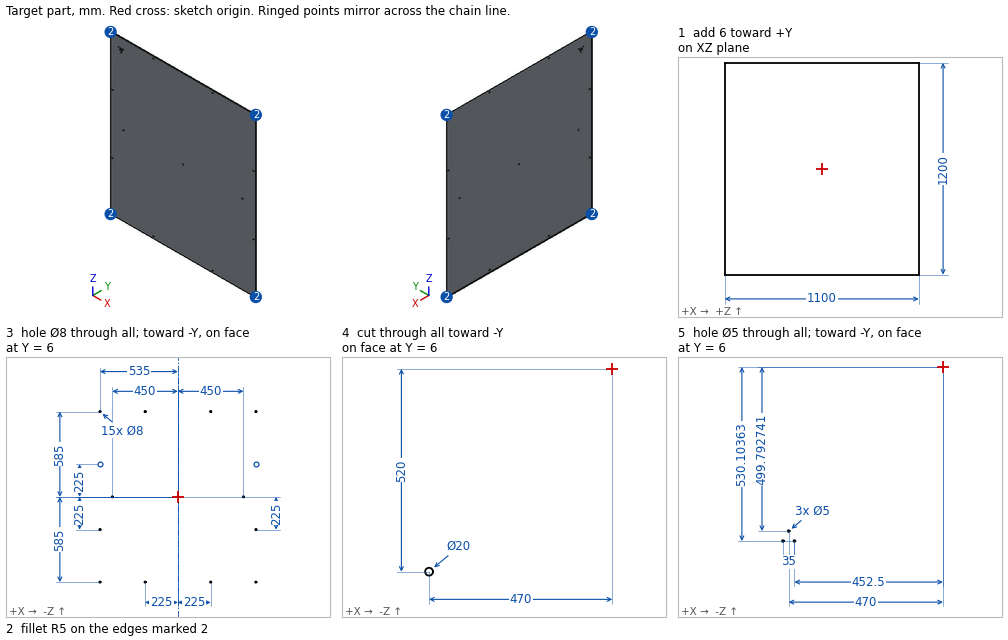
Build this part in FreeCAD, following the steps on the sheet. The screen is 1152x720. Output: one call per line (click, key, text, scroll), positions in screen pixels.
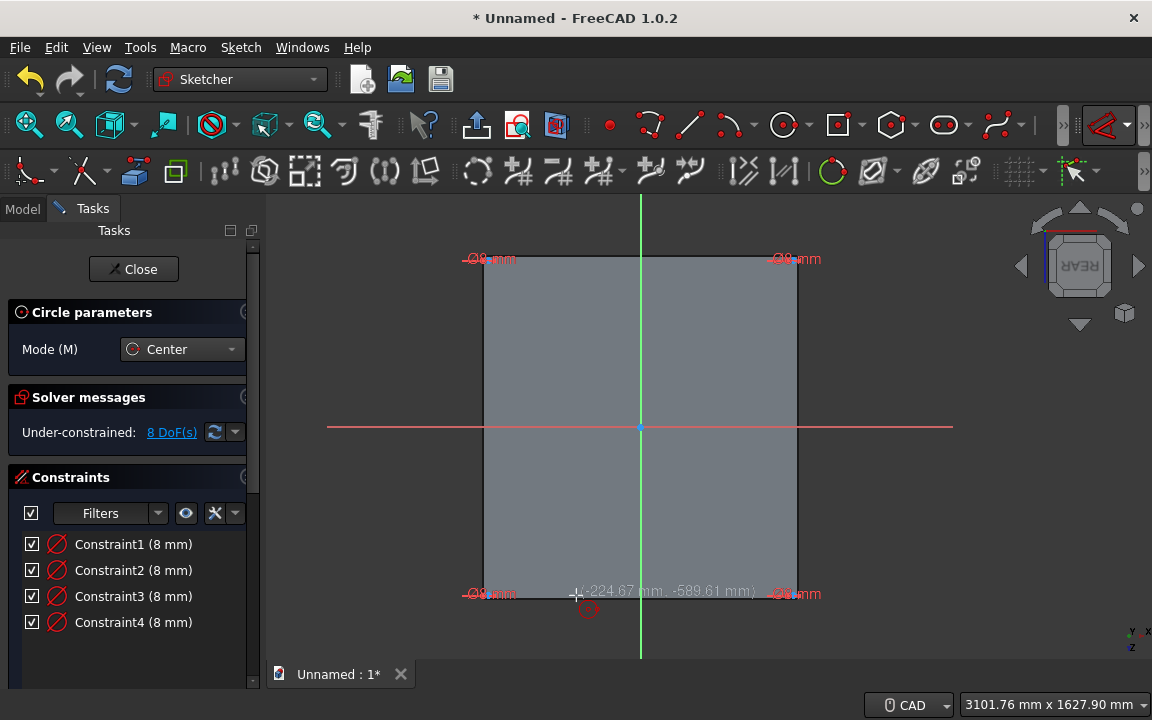
click(576, 595)
move(577, 594)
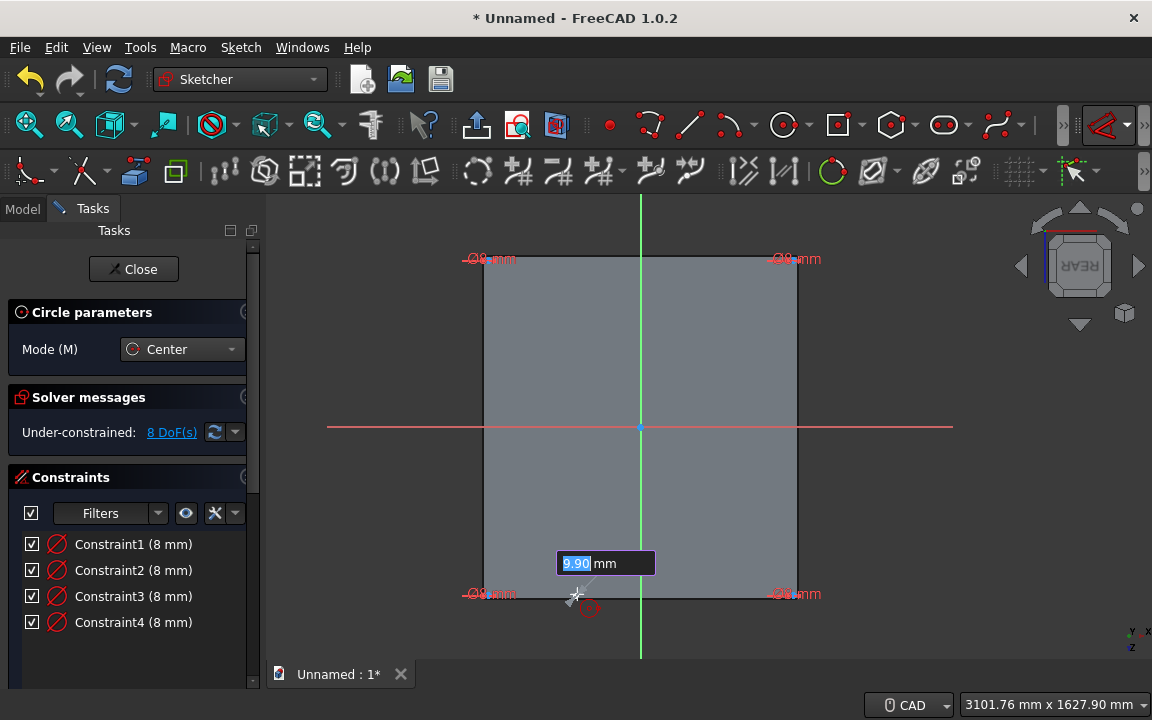
text(8)
key(Return)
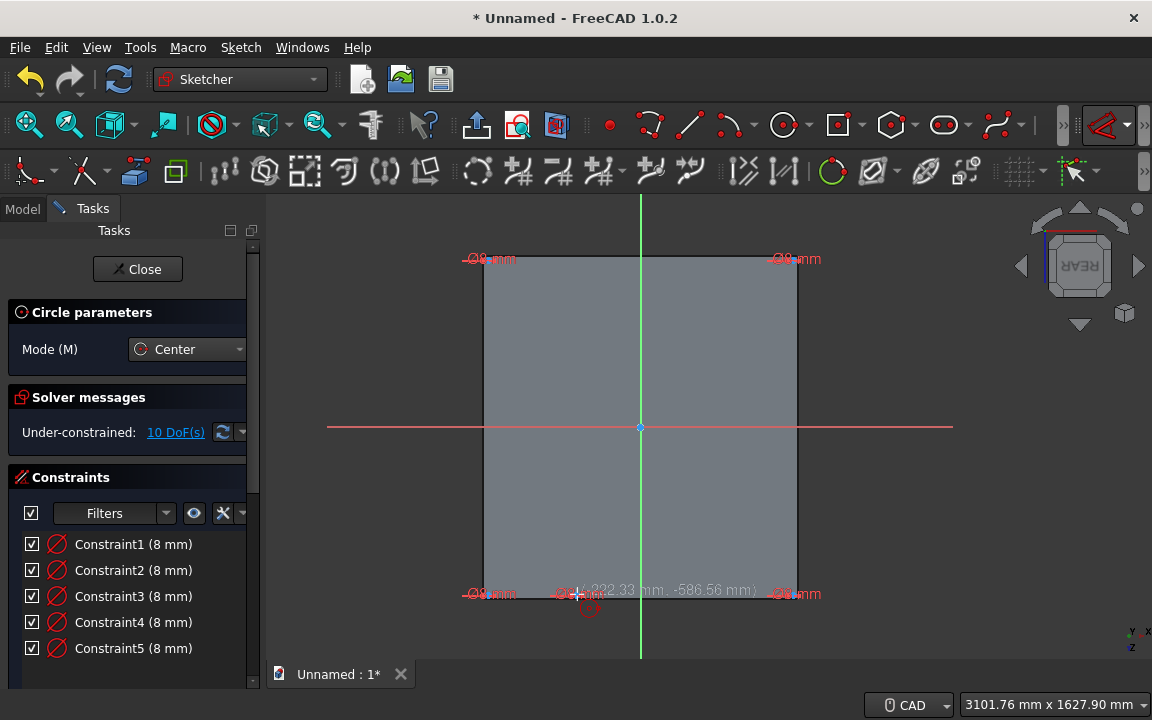
scroll(705, 595, up, 15)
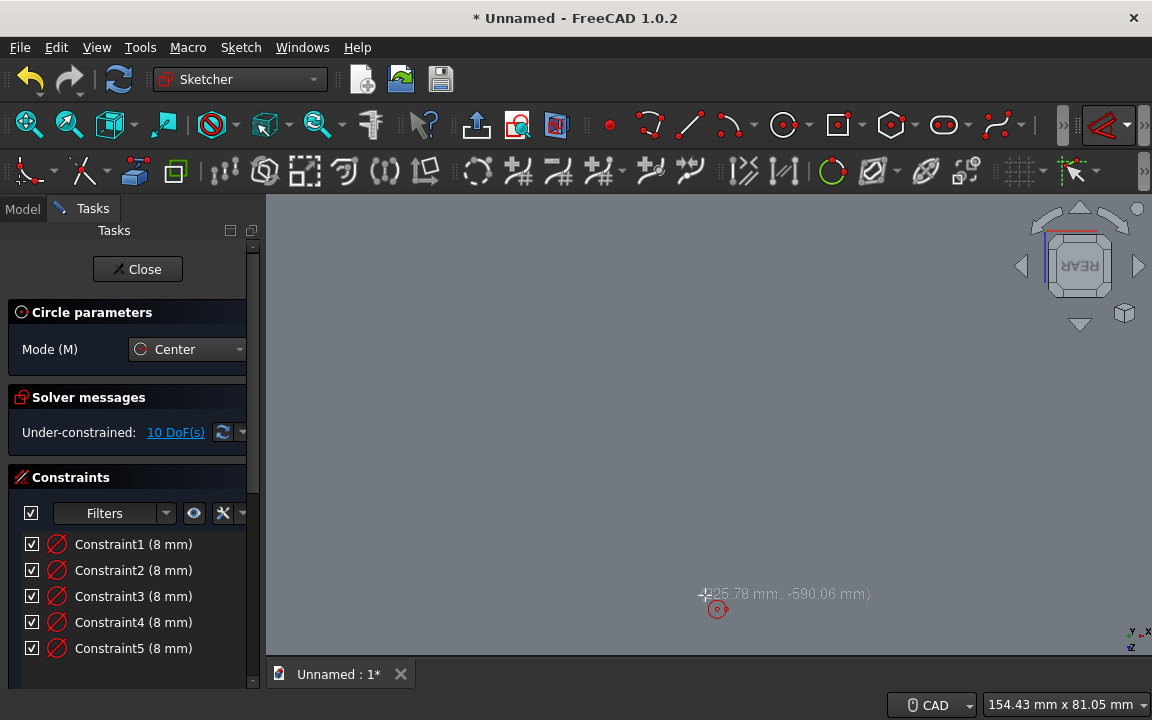
scroll(705, 595, down, 15)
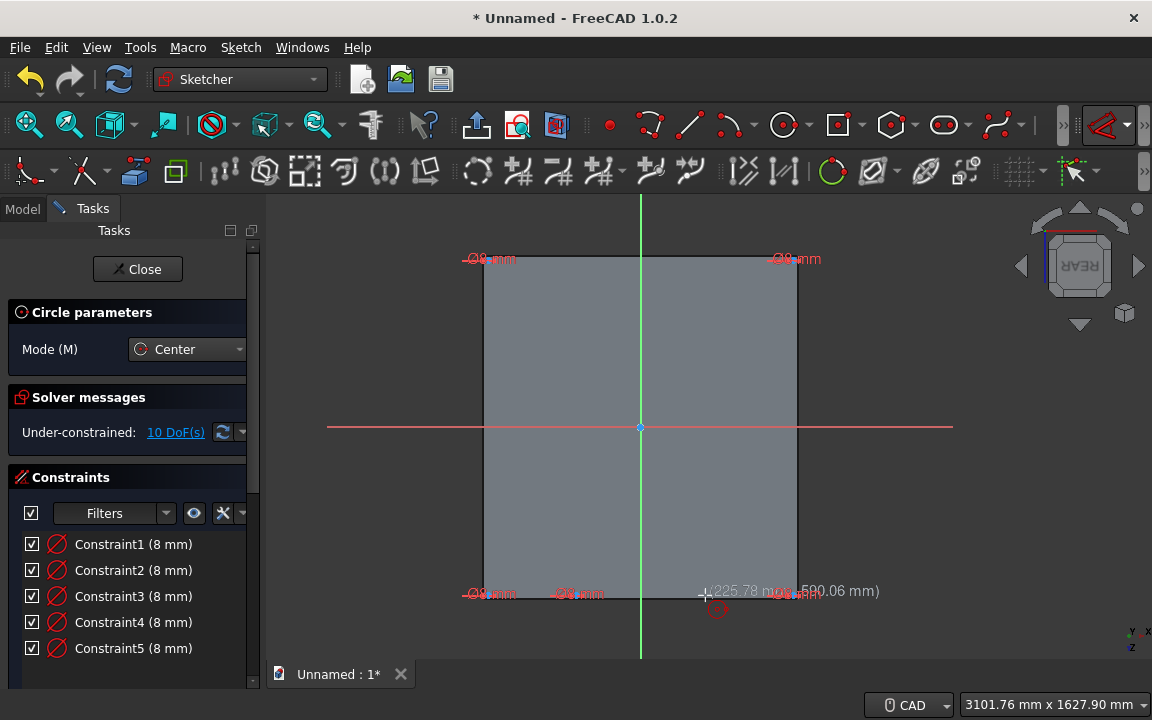
click(705, 595)
move(706, 594)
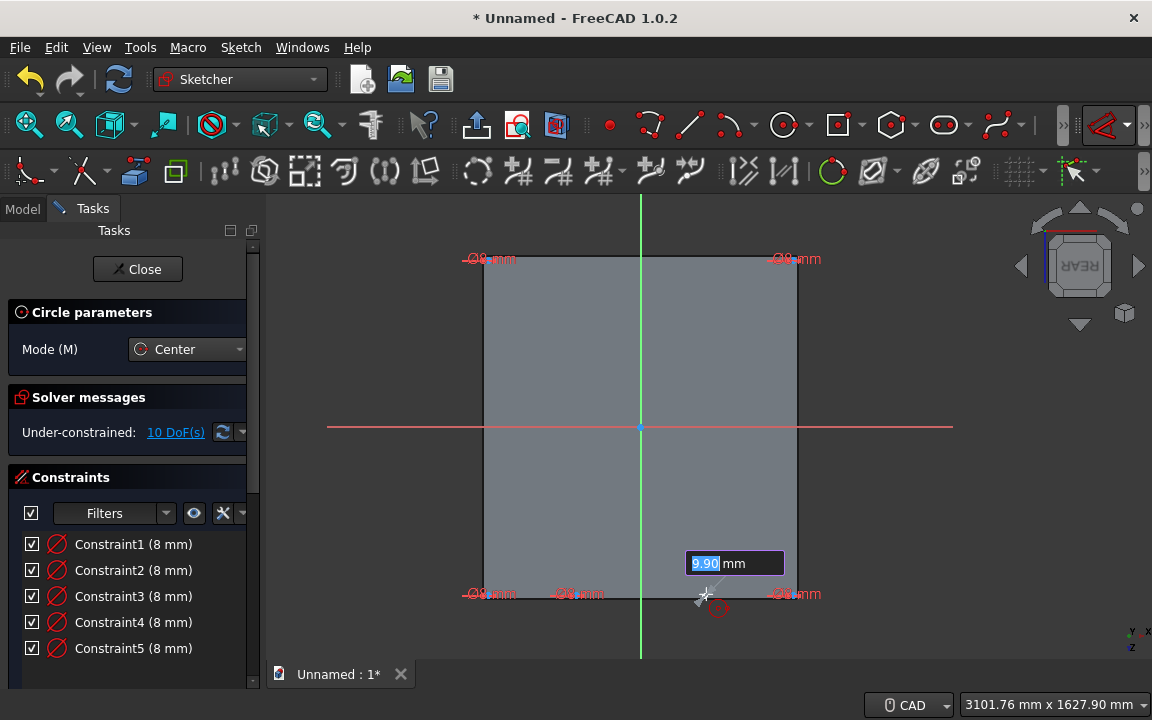
text(8)
key(Return)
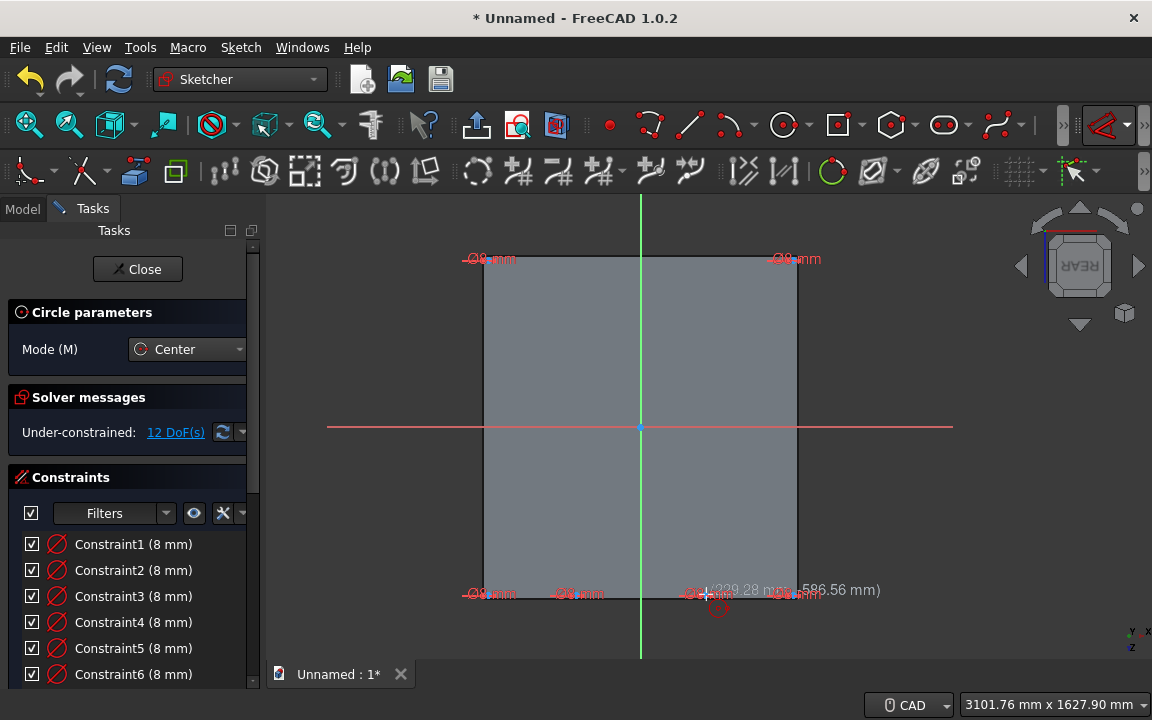
scroll(641, 427, up, 15)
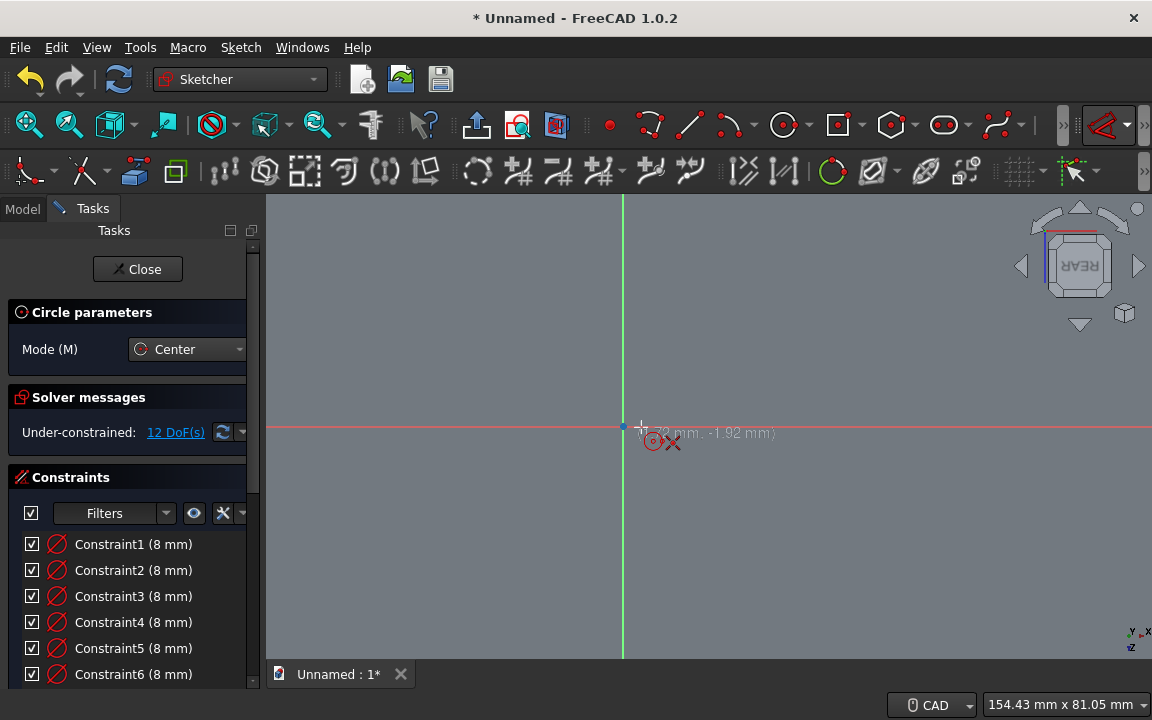
scroll(641, 426, down, 15)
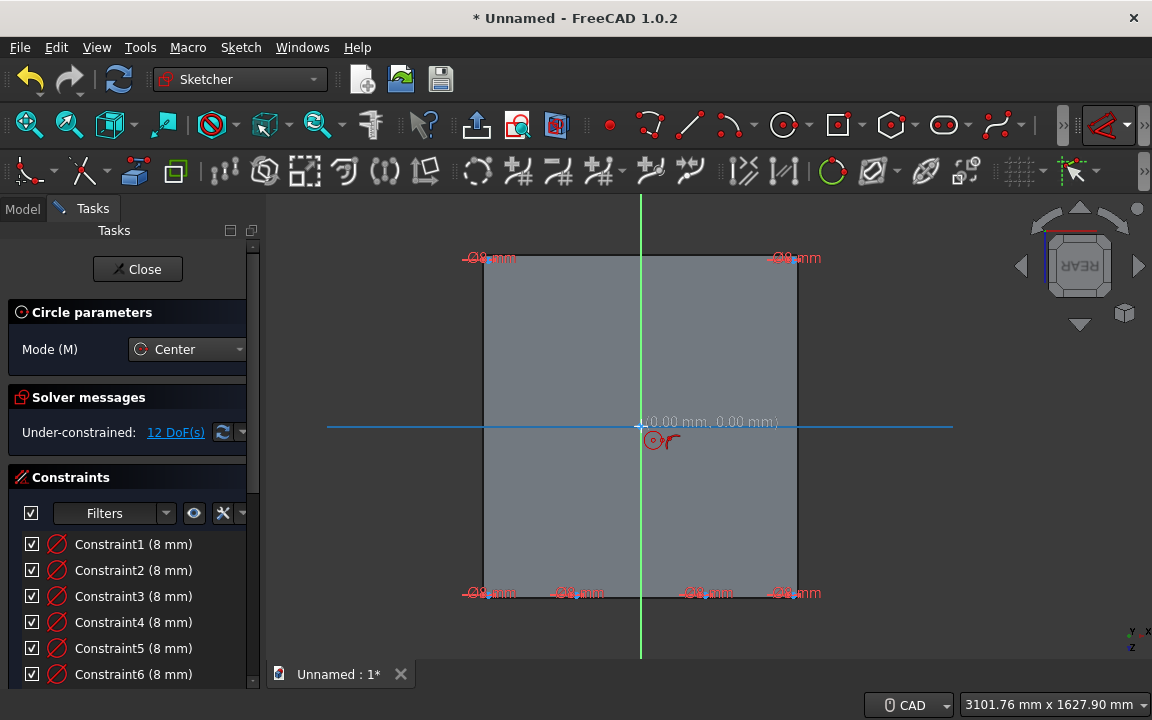
click(641, 427)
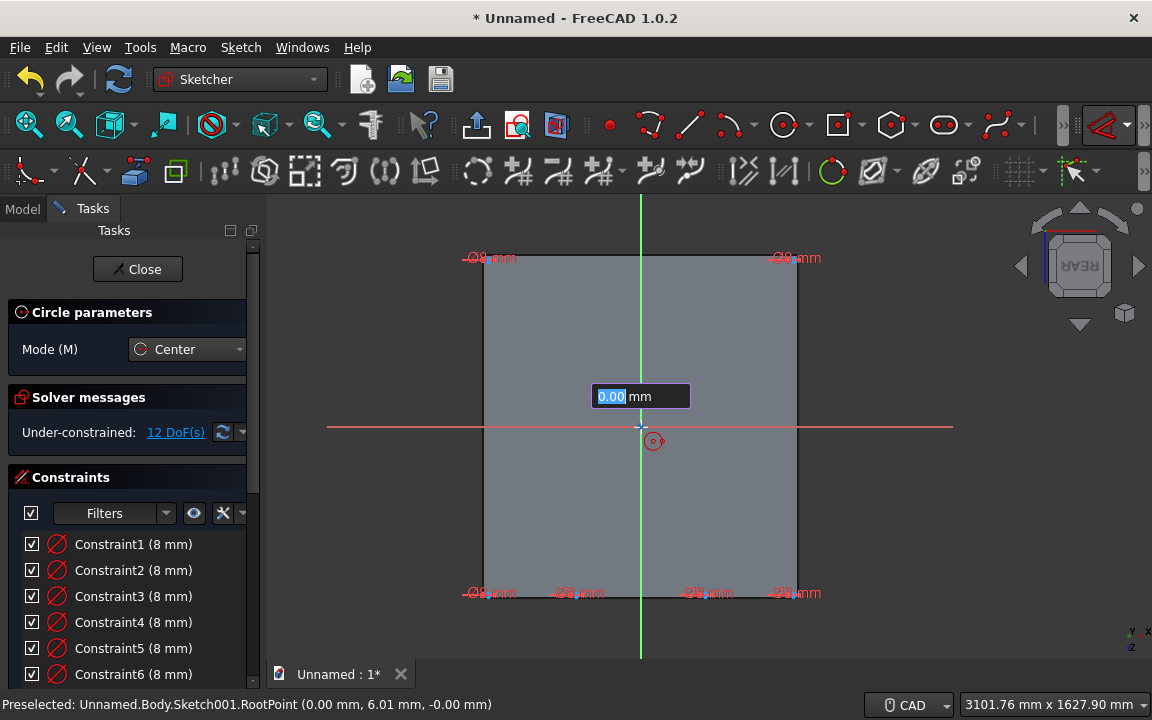
scroll(641, 426, up, 15)
move(639, 410)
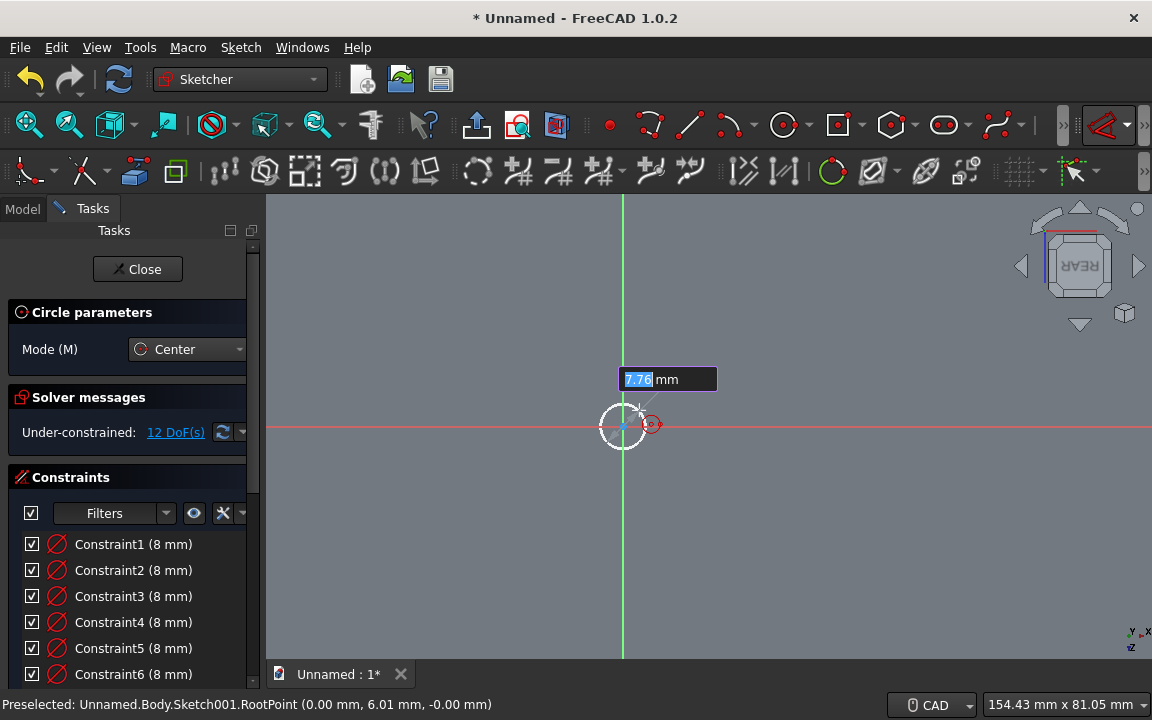
text(8)
key(Return)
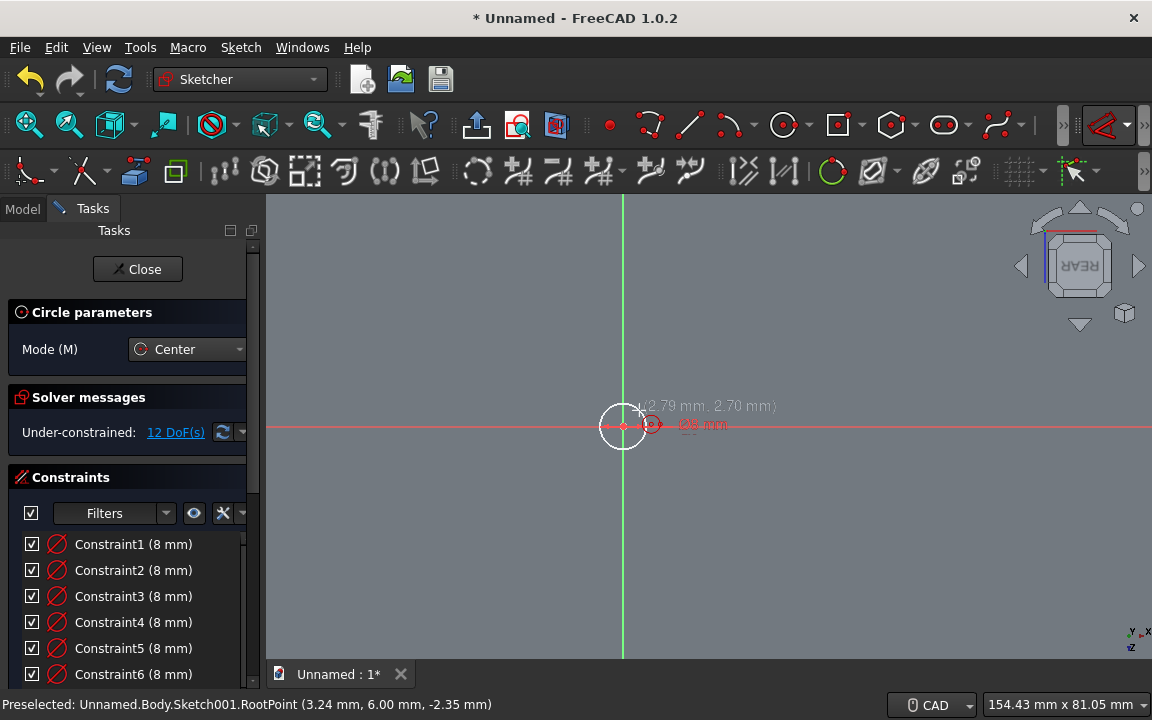
scroll(641, 426, down, 15)